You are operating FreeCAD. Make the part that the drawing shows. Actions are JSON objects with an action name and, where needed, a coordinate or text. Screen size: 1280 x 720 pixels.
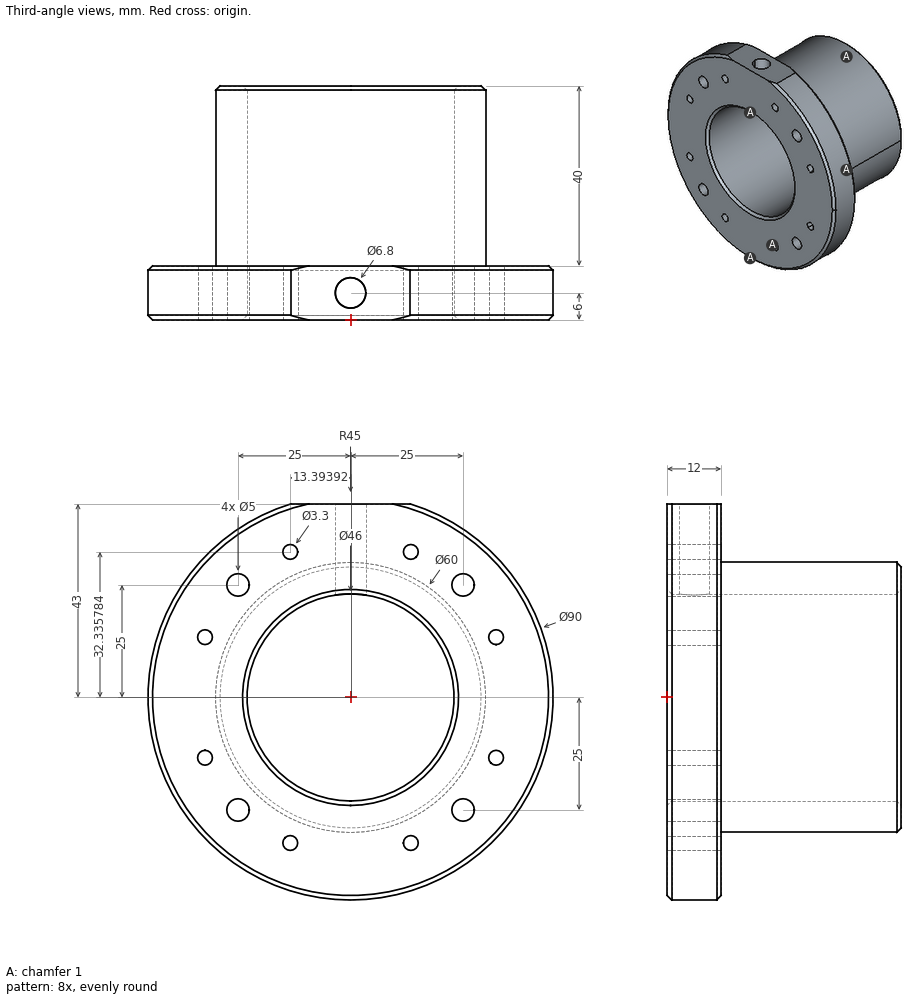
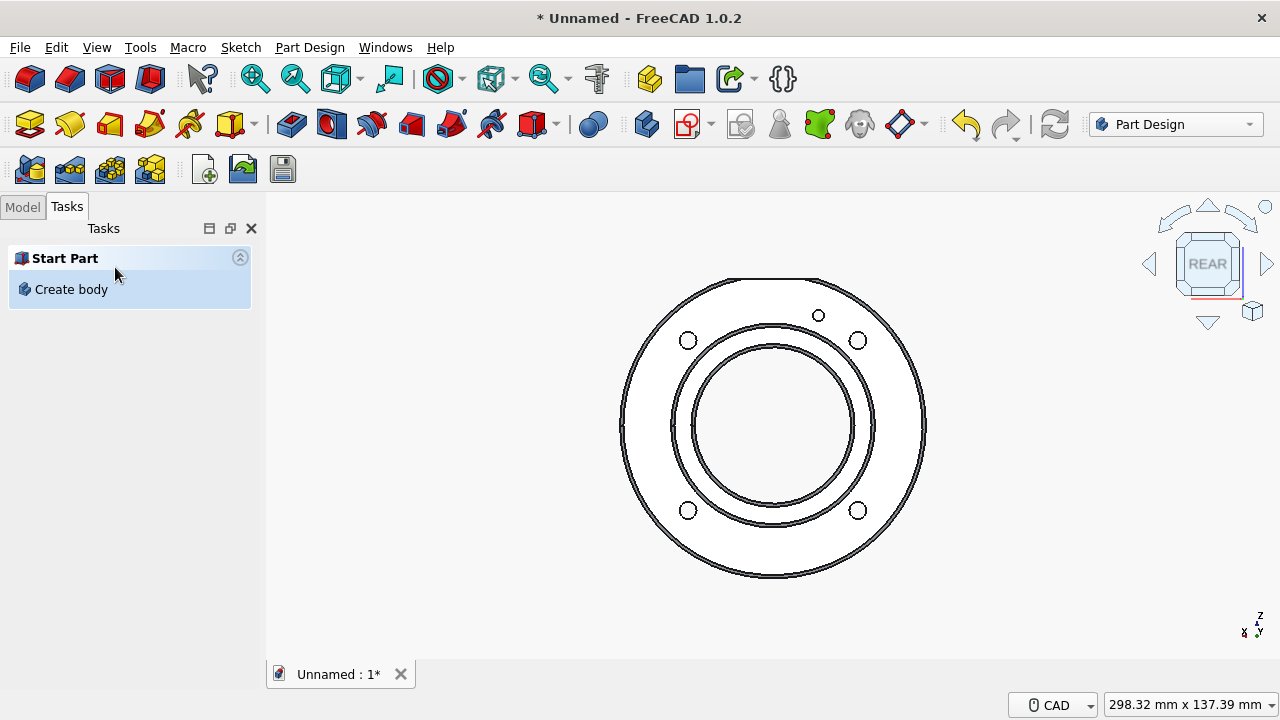
{"action": "left_click", "coordinate": [23, 206]}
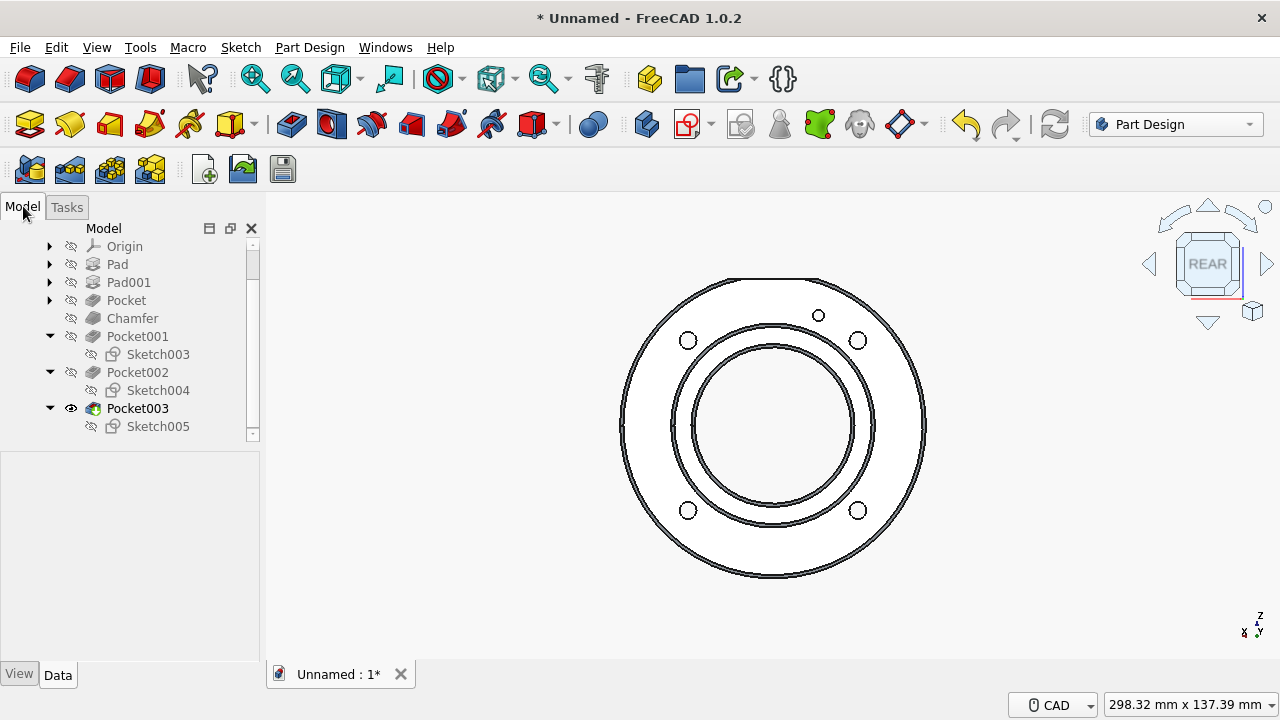
{"action": "left_click", "coordinate": [116, 372]}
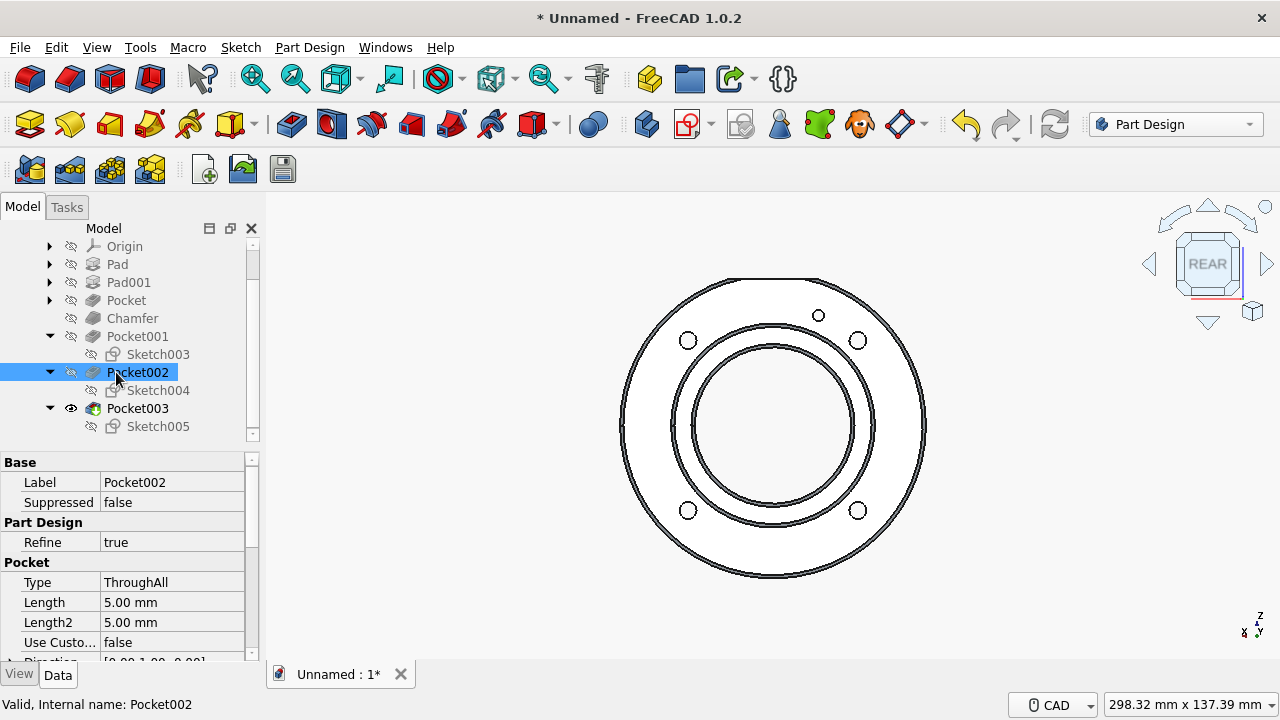
{"action": "left_click", "coordinate": [110, 170]}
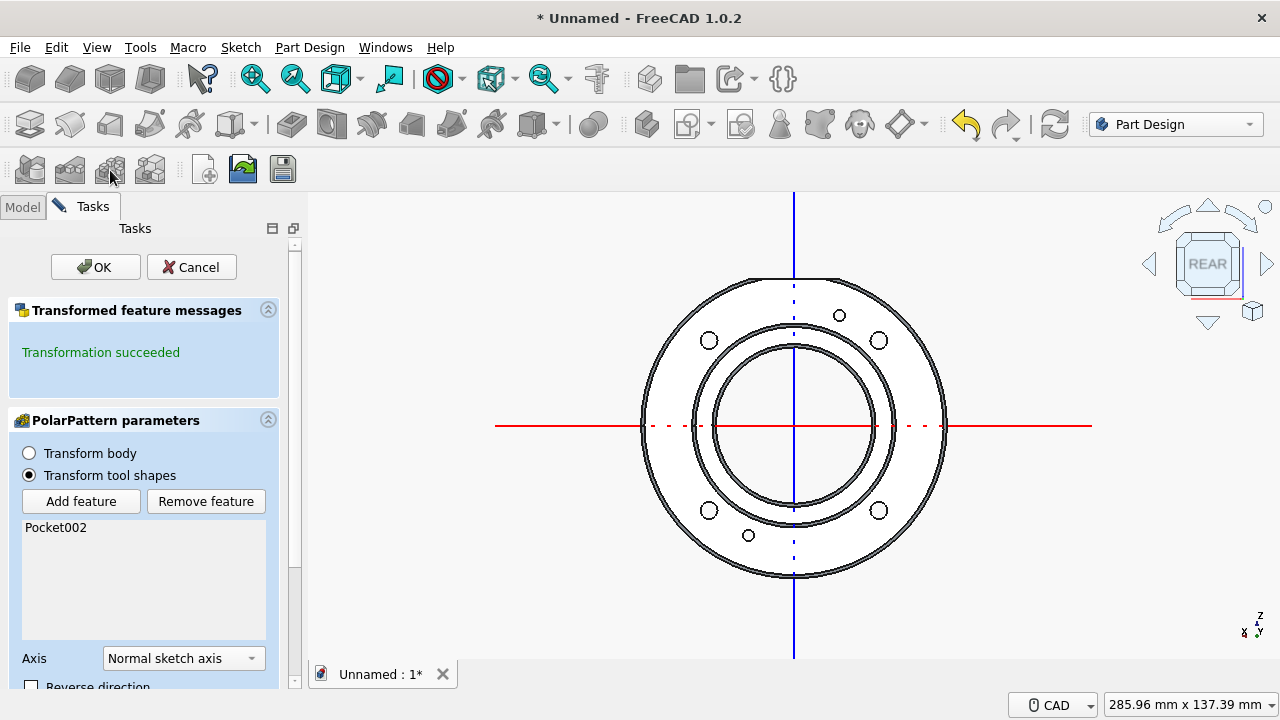
{"action": "left_click", "coordinate": [184, 658]}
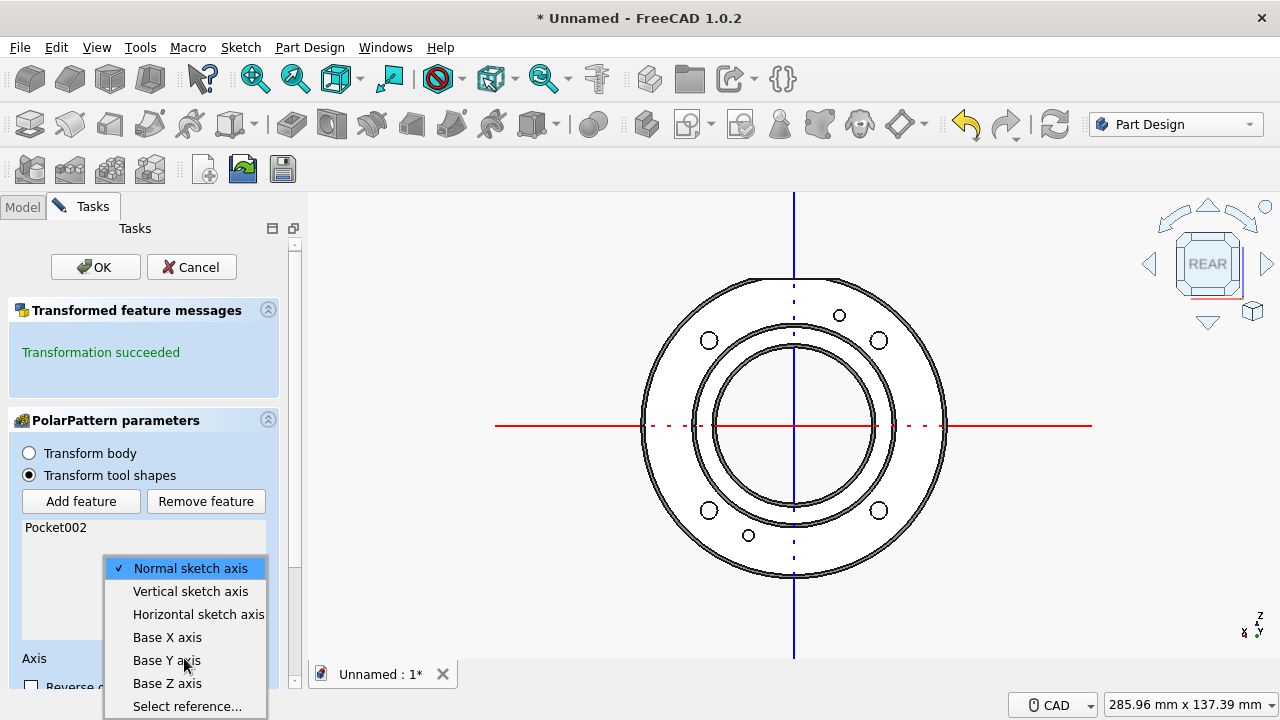
{"action": "left_click", "coordinate": [184, 660]}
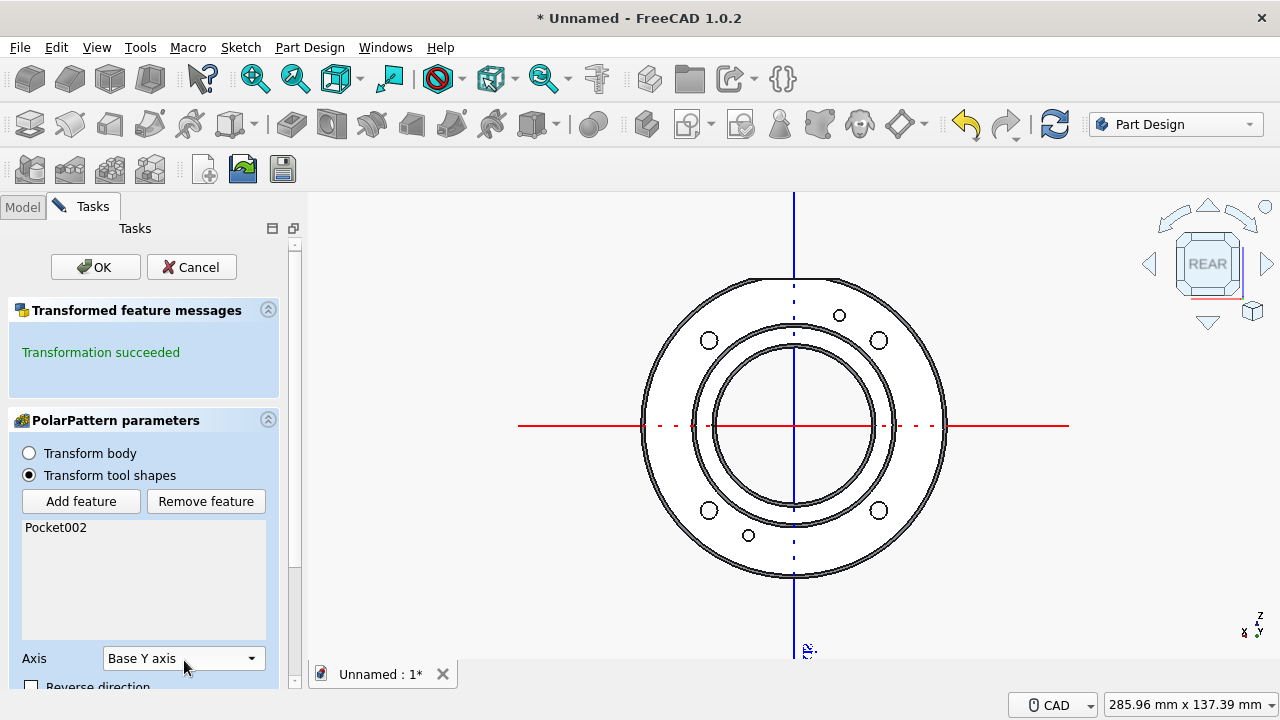
{"action": "scroll", "coordinate": [295, 463], "scroll_direction": "down", "scroll_amount": 3}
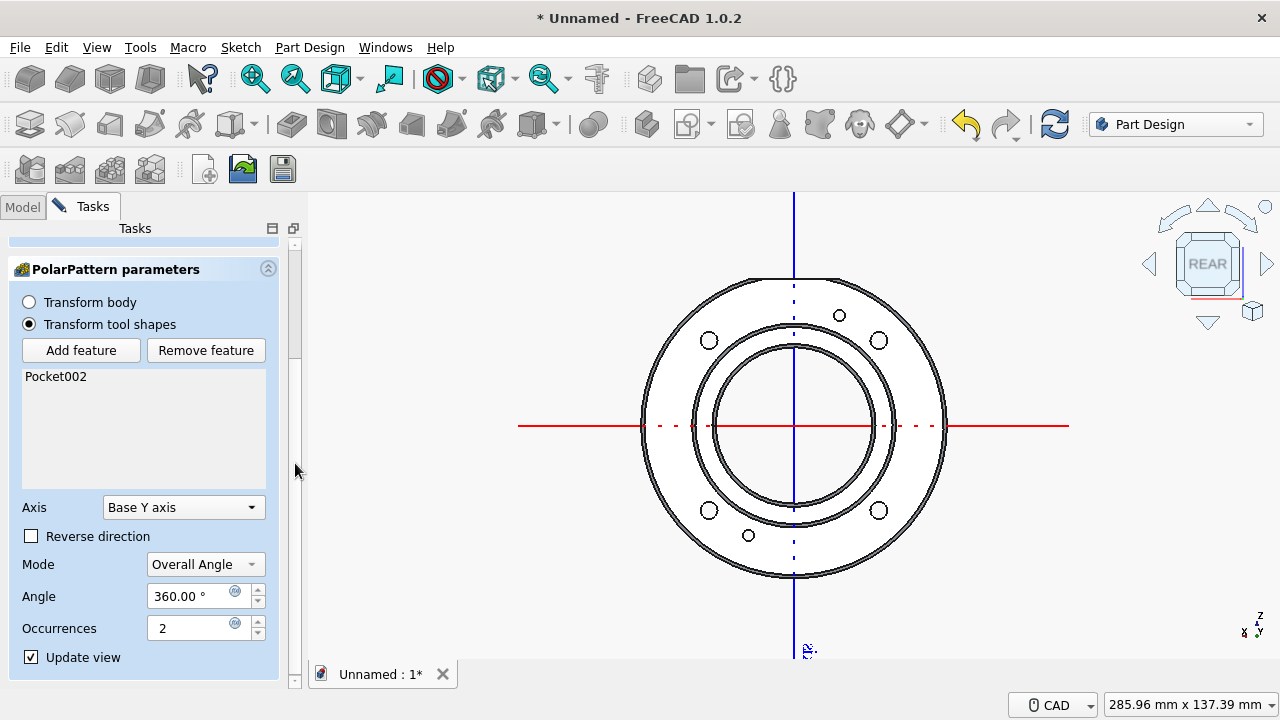
{"action": "triple_click", "coordinate": [198, 628]}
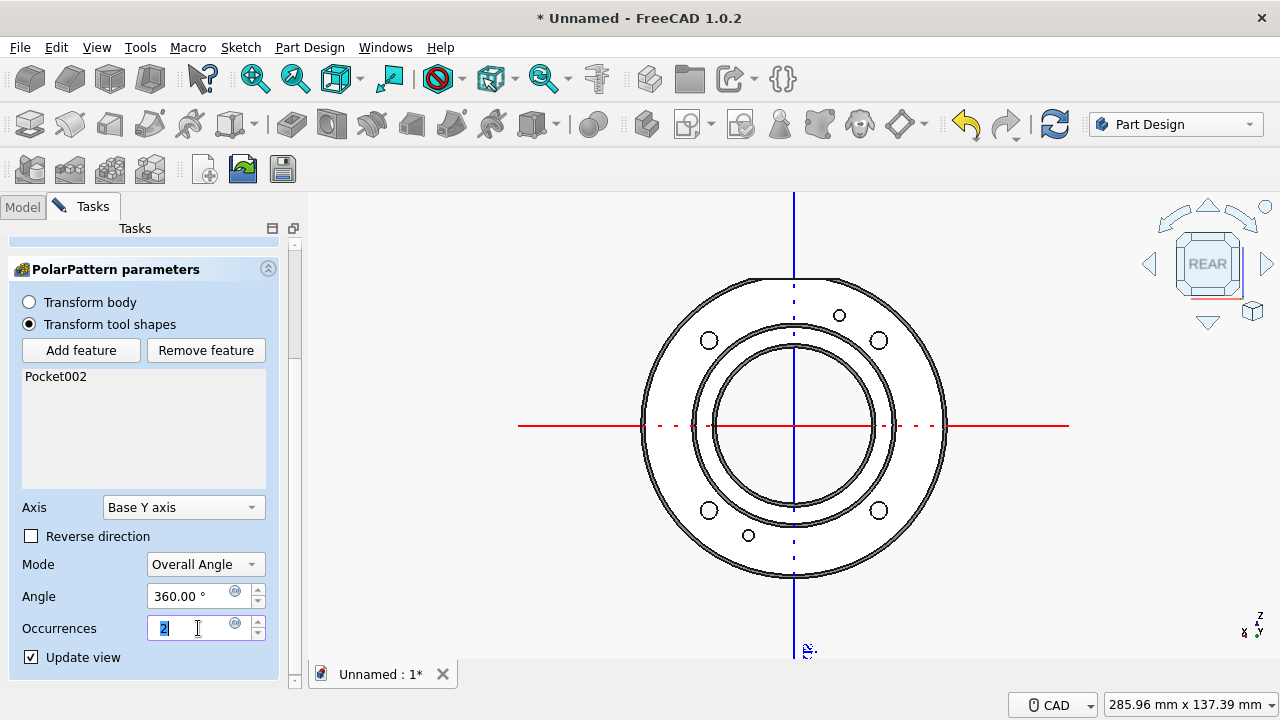
{"action": "type", "text": "8"}
{"action": "key", "text": "Tab"}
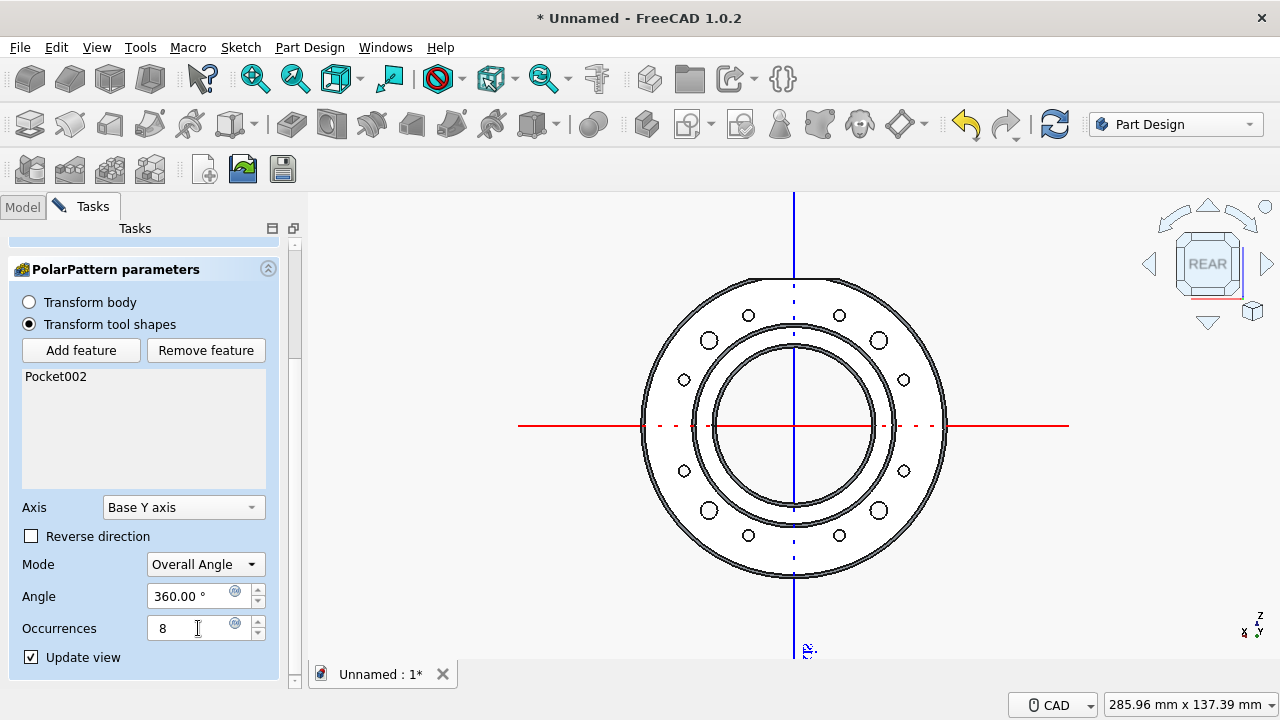
{"action": "scroll", "coordinate": [295, 463], "scroll_direction": "up", "scroll_amount": 4}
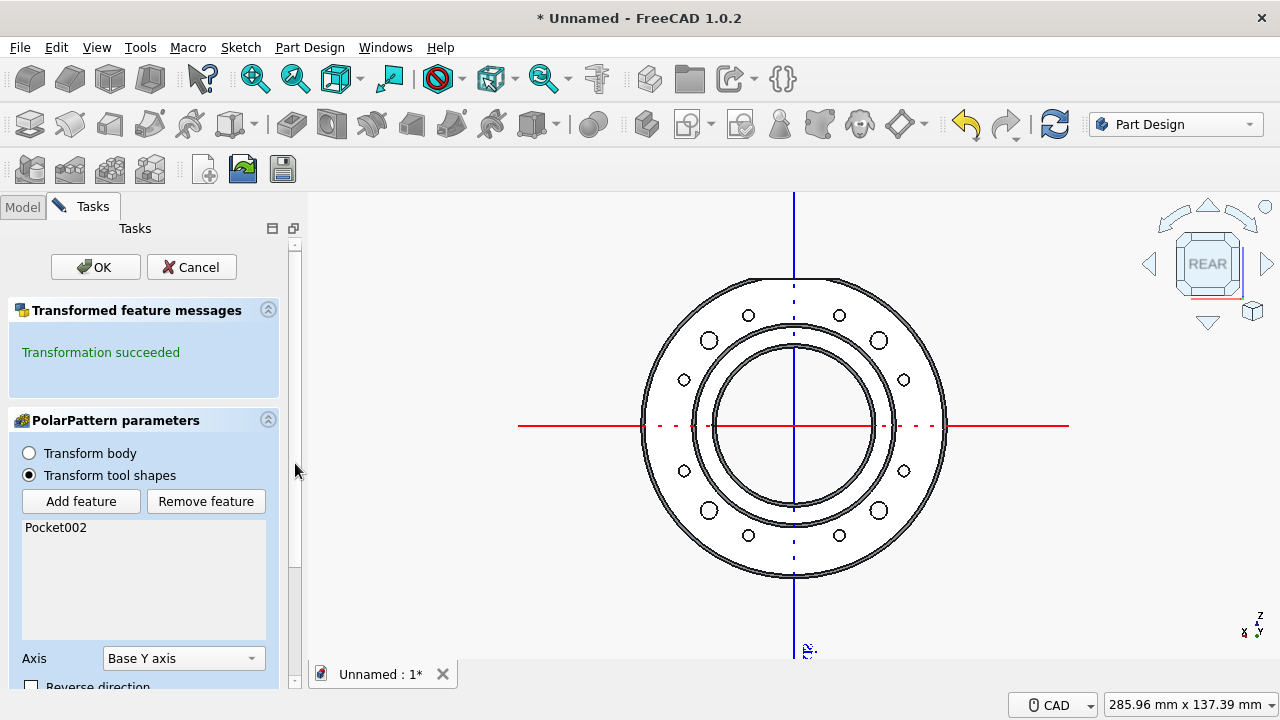
{"action": "left_click", "coordinate": [96, 267]}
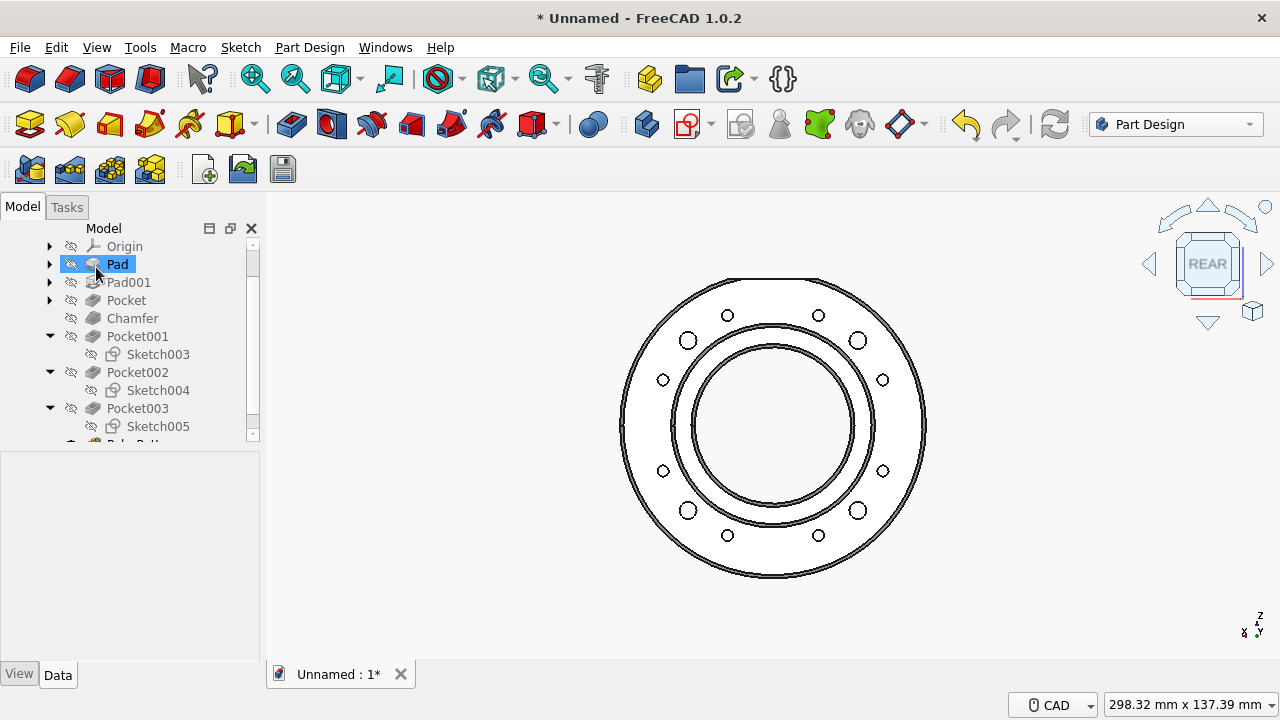
{"action": "key", "text": "0"}